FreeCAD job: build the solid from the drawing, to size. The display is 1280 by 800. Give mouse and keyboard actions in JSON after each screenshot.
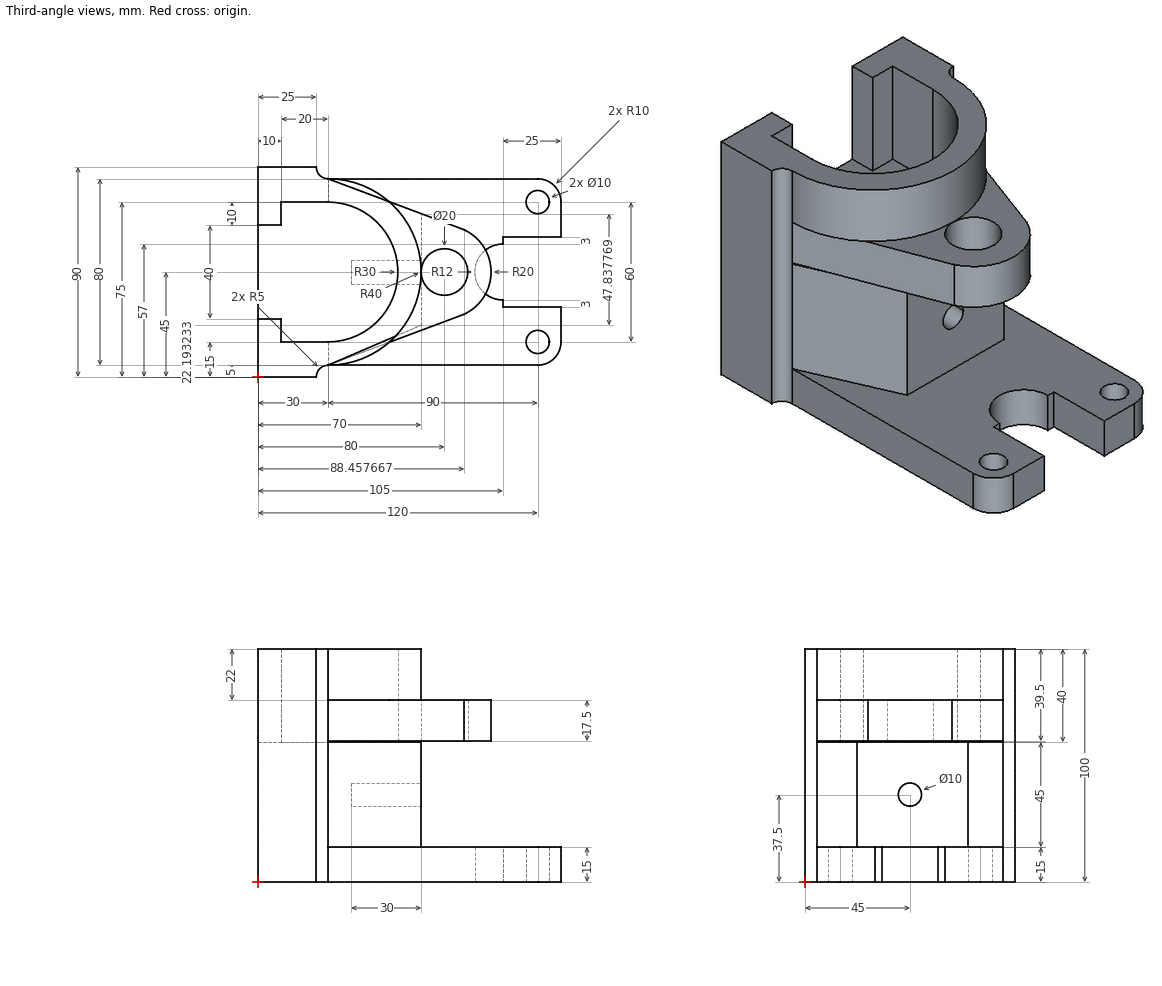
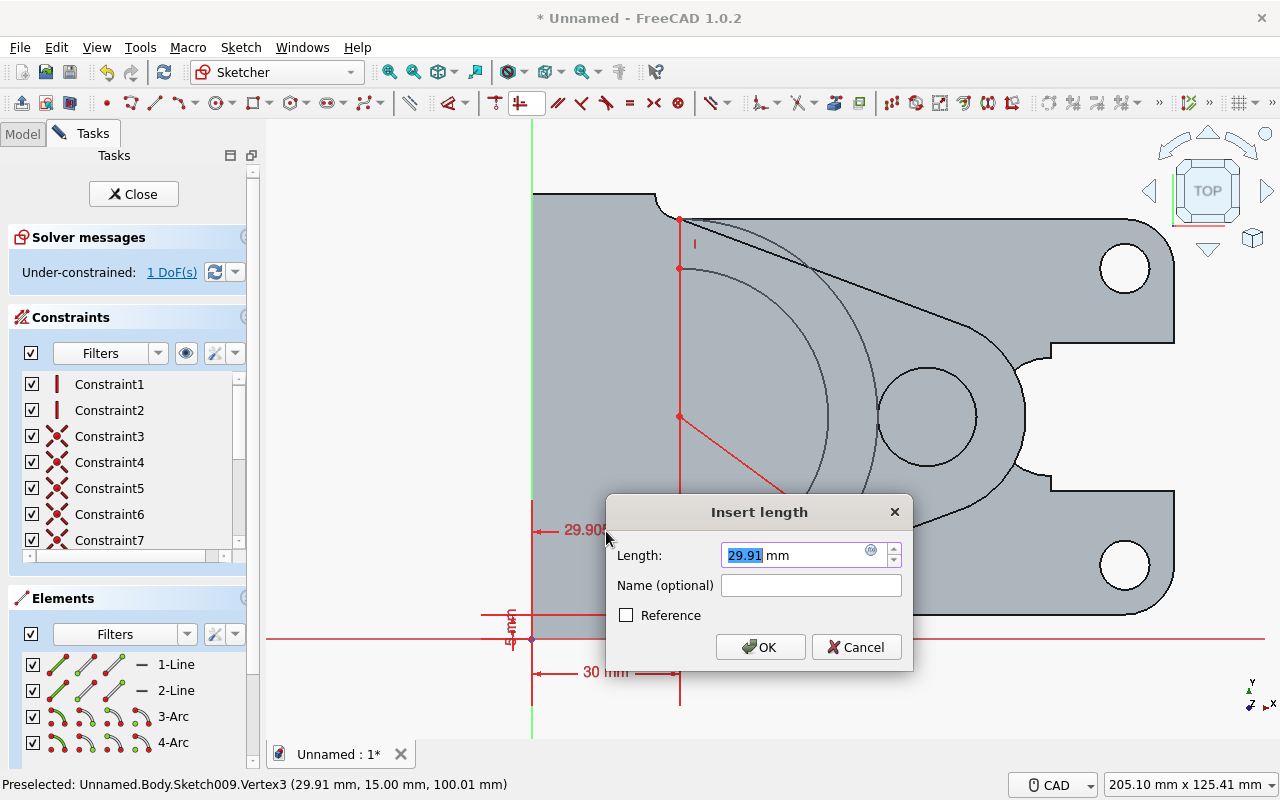
{"action": "type", "text": "30"}
{"action": "key", "text": "Return"}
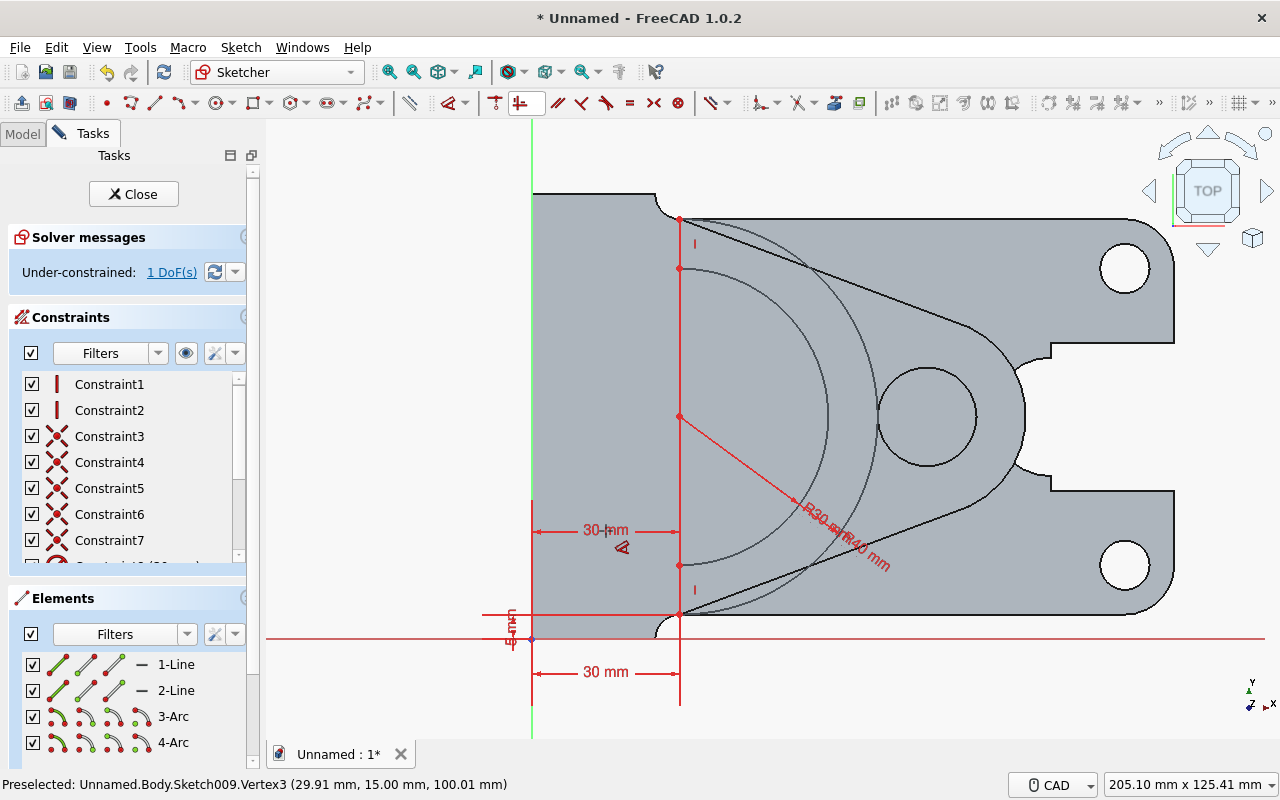
{"action": "left_click", "coordinate": [680, 417]}
{"action": "left_click", "coordinate": [606, 383]}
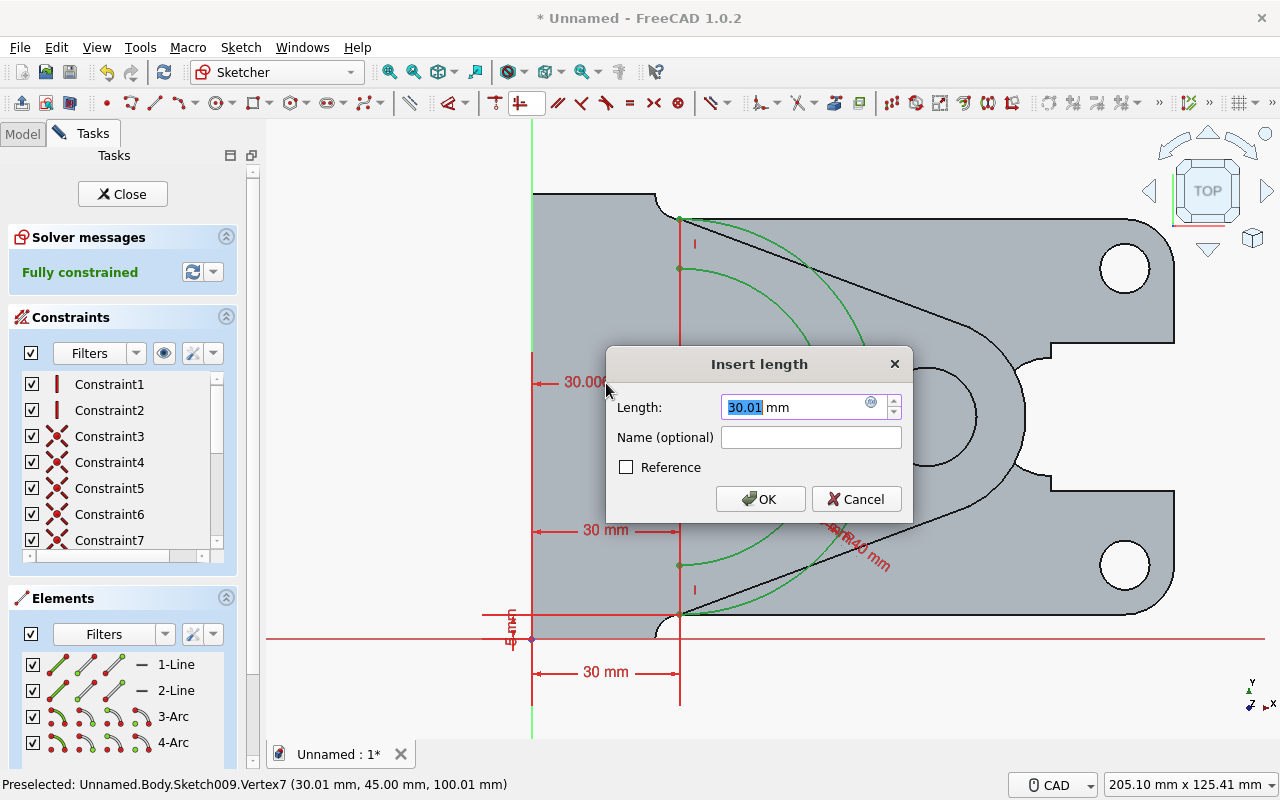
{"action": "type", "text": "30"}
{"action": "key", "text": "Return"}
{"action": "key", "text": "Escape"}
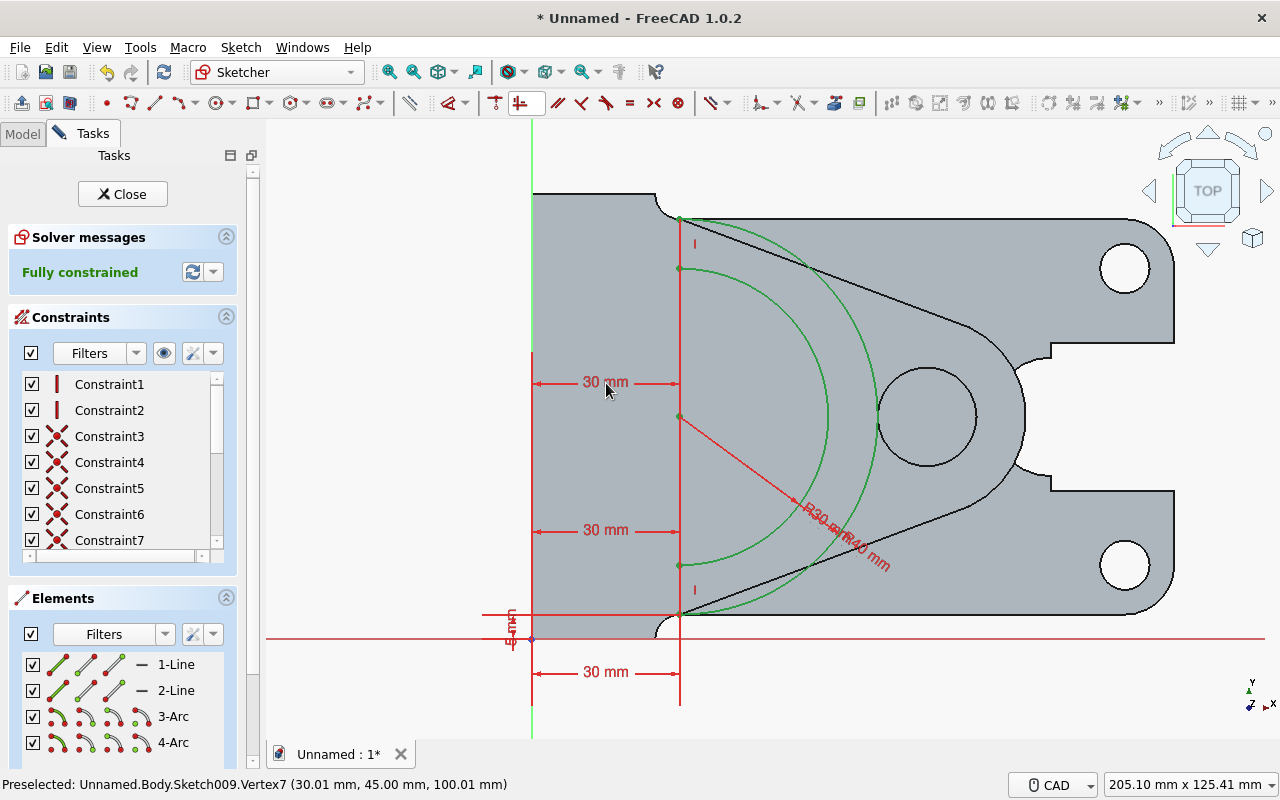
{"action": "left_click", "coordinate": [123, 194]}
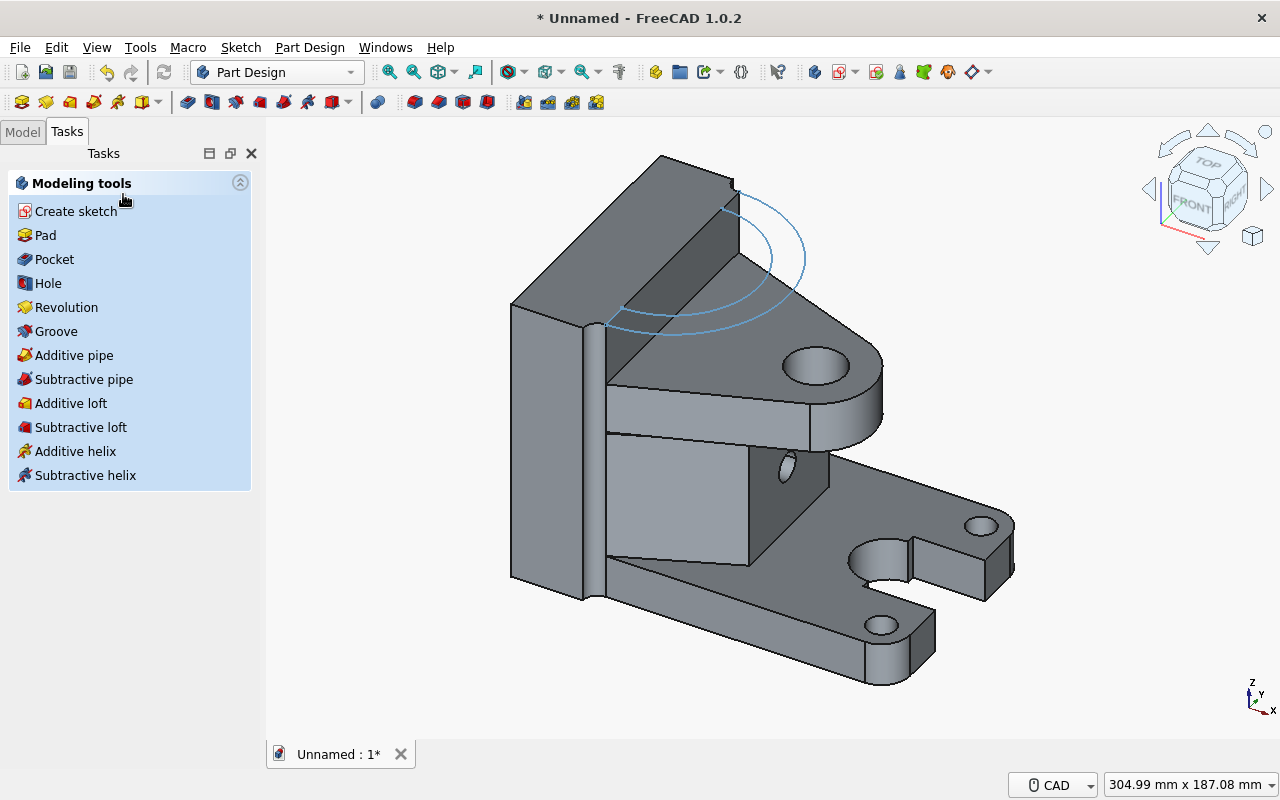
{"action": "left_click", "coordinate": [22, 102]}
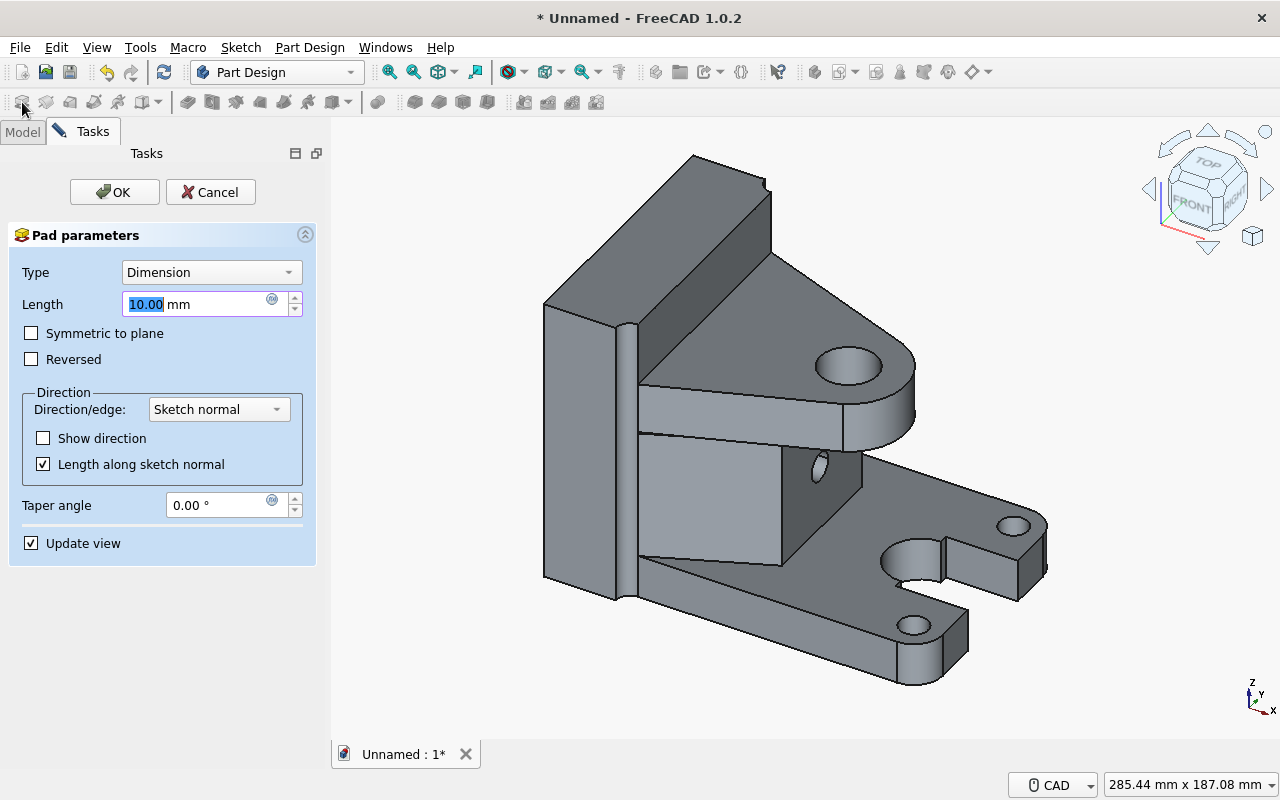
{"action": "type", "text": "22"}
{"action": "key", "text": "Tab"}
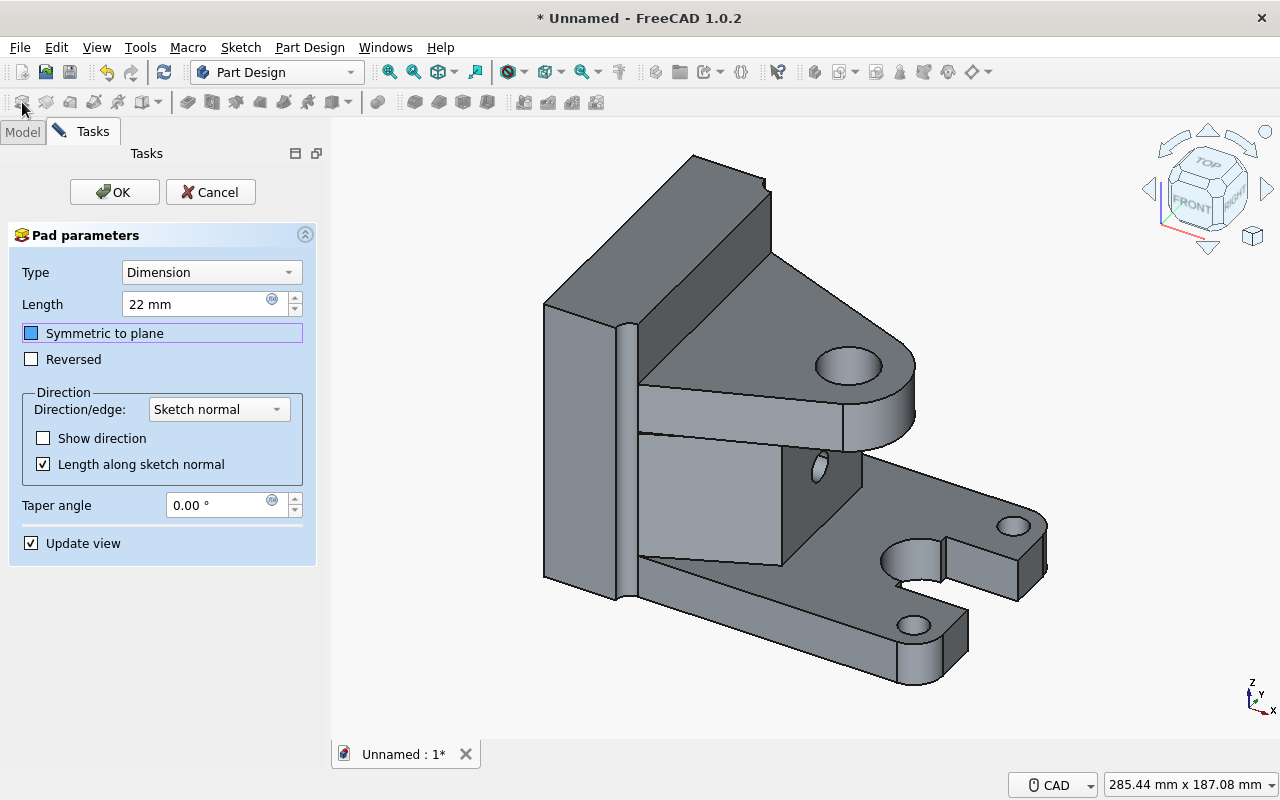
{"action": "left_click", "coordinate": [30, 359]}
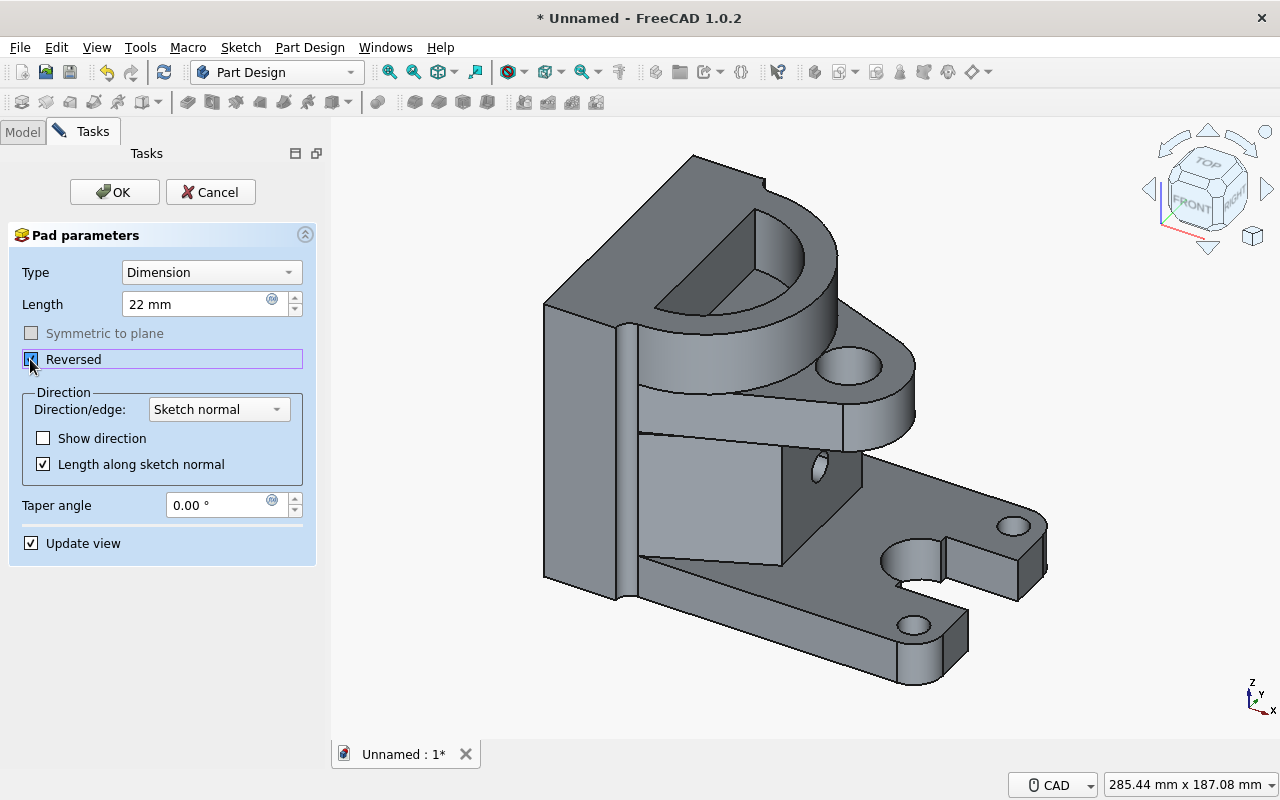
{"action": "left_click", "coordinate": [115, 192]}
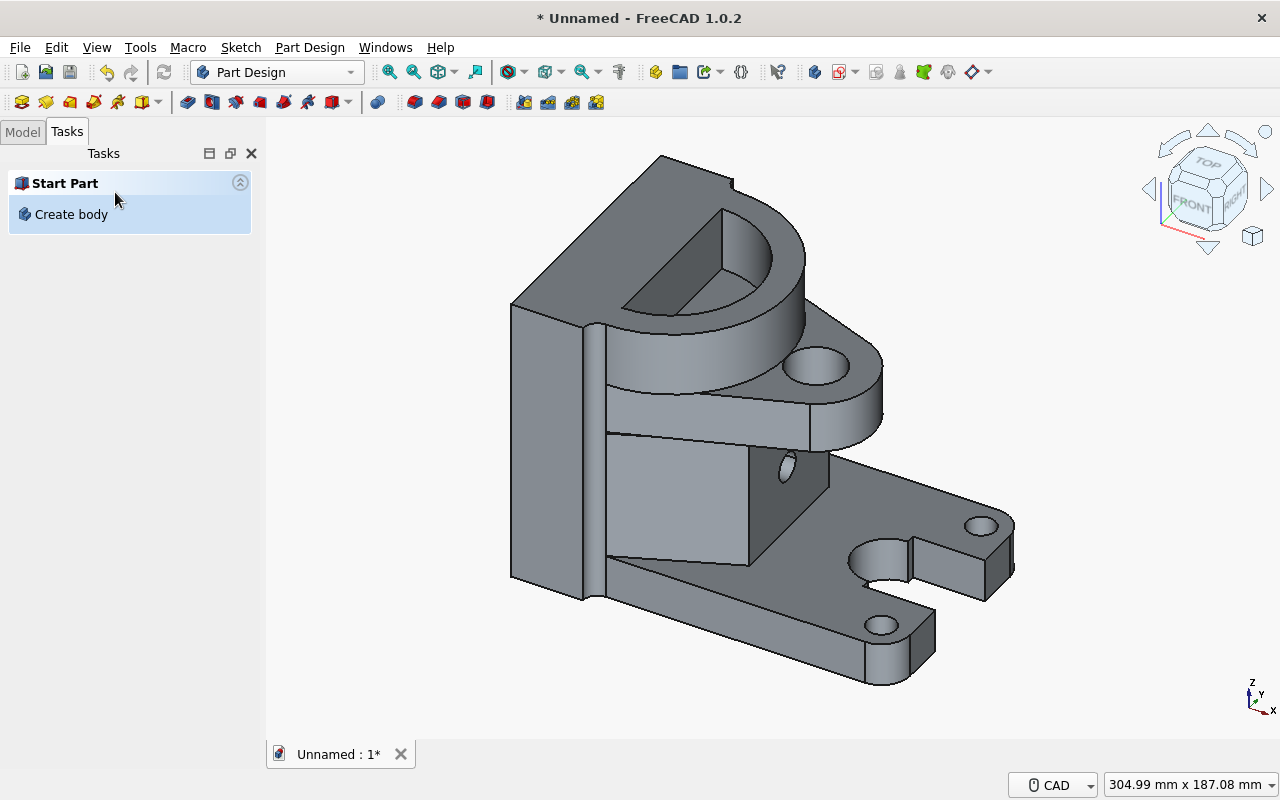
{"action": "left_click", "coordinate": [672, 201]}